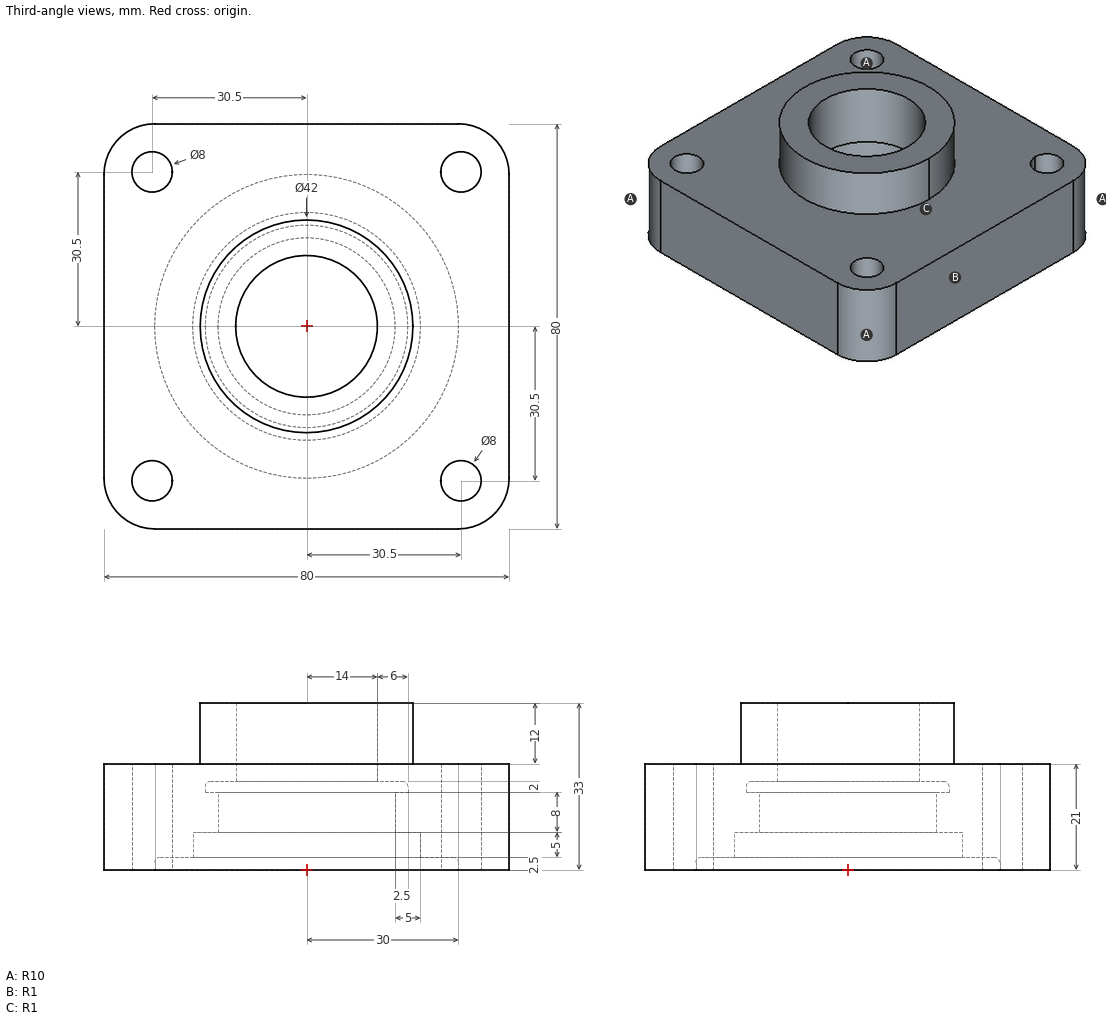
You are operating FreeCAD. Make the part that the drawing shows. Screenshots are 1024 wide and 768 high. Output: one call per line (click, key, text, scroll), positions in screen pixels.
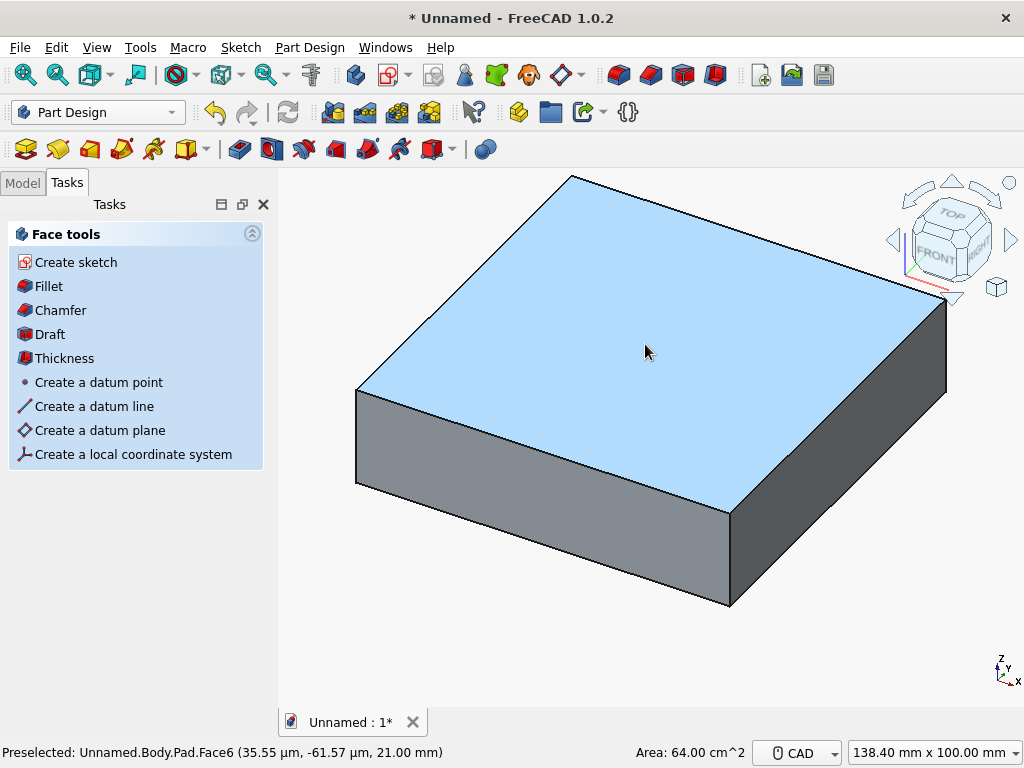
click(388, 76)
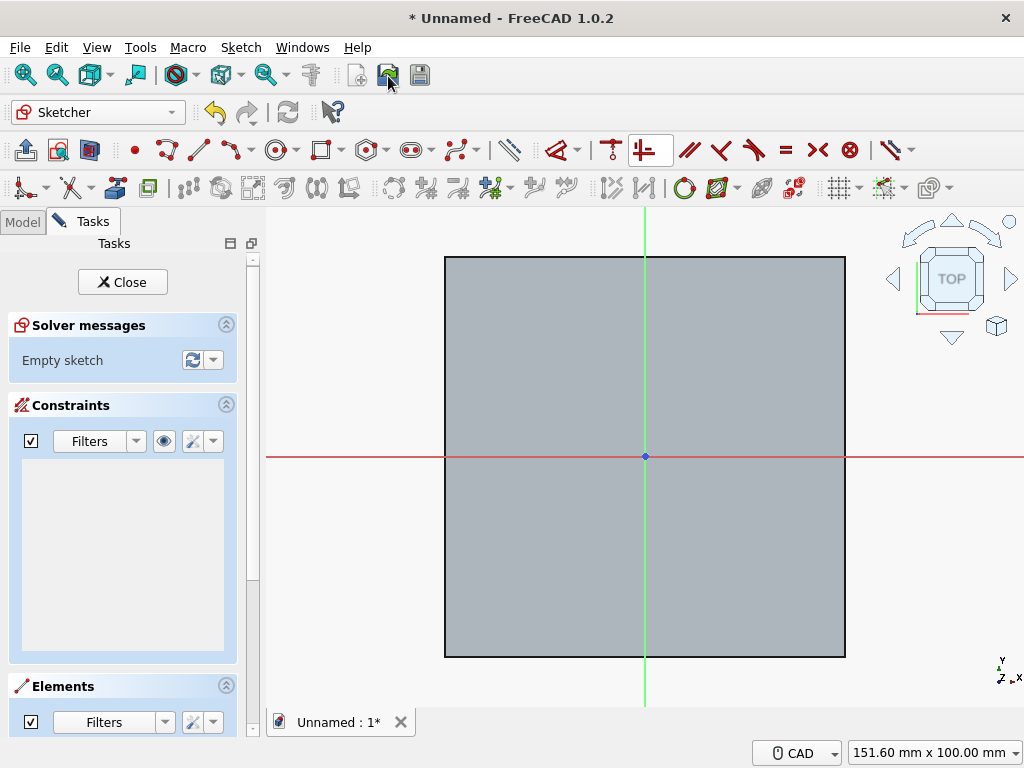
scroll(784, 457, up, 2)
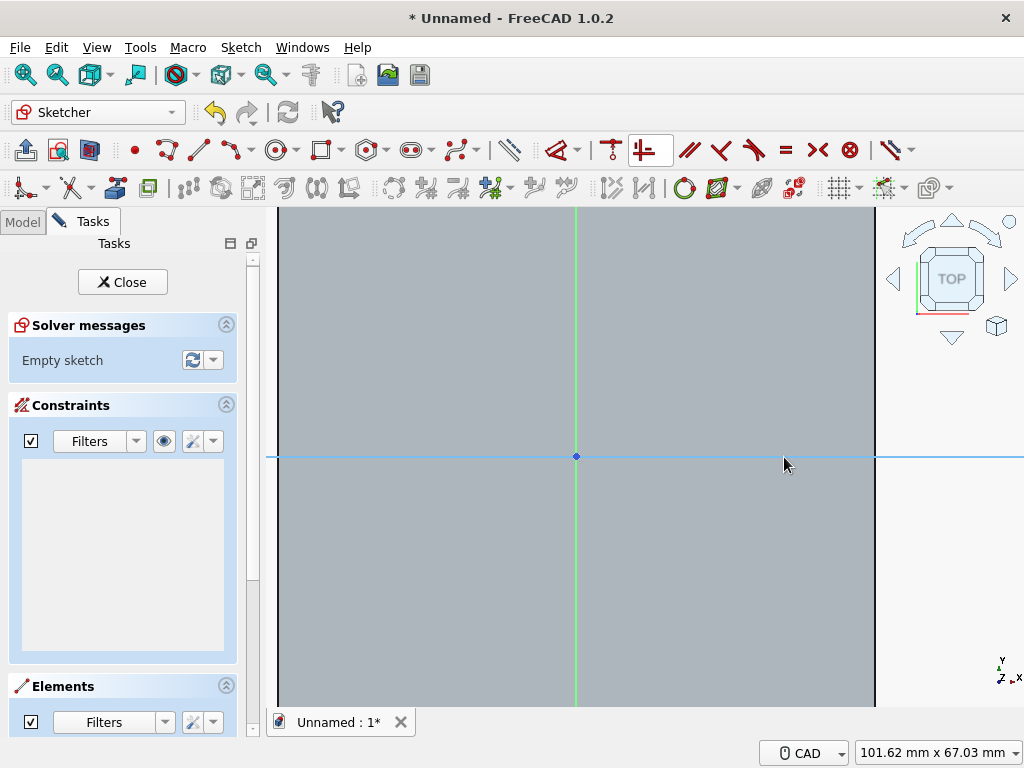
click(276, 150)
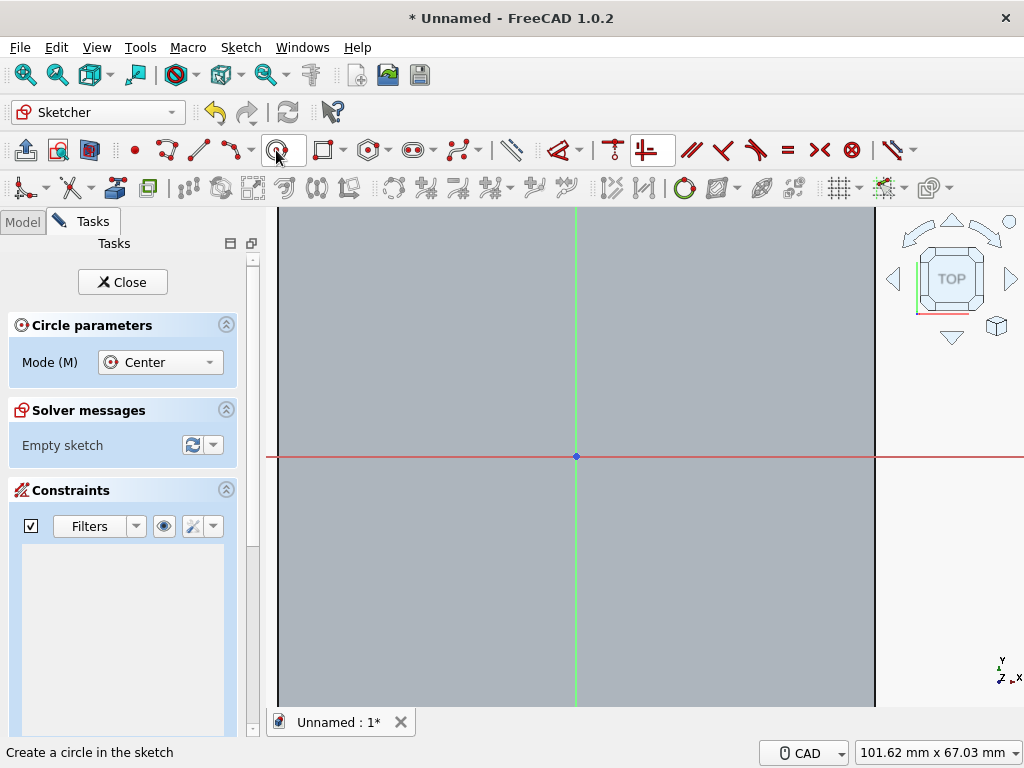
click(576, 457)
move(687, 346)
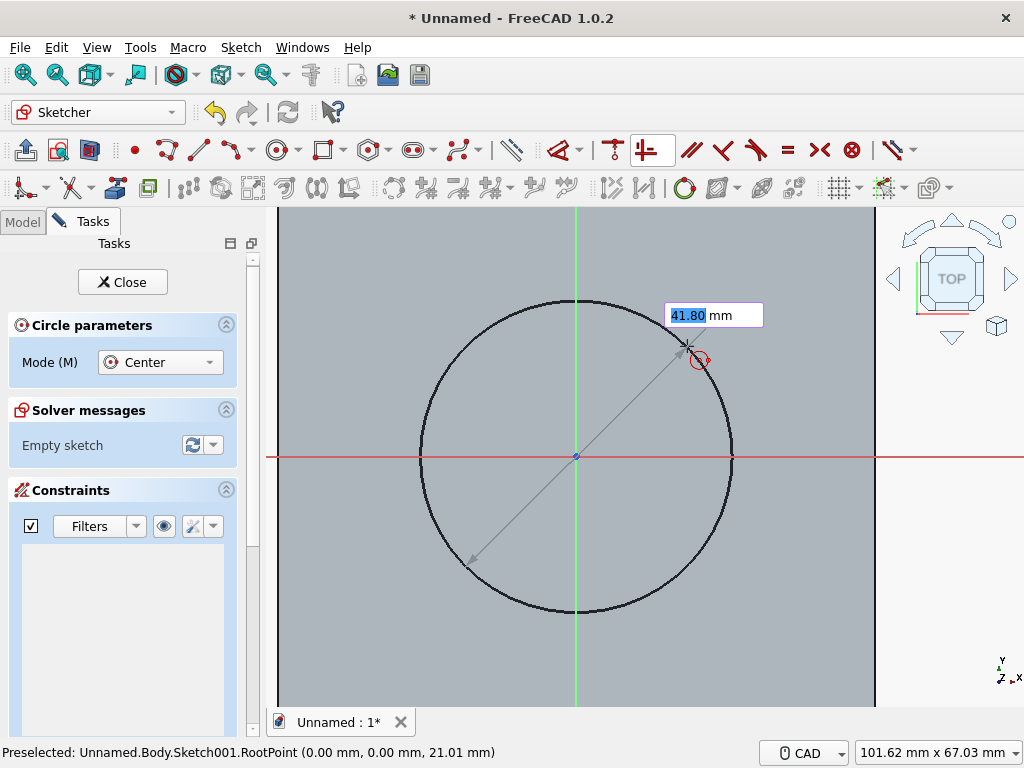
text(42)
key(Return)
key(Escape)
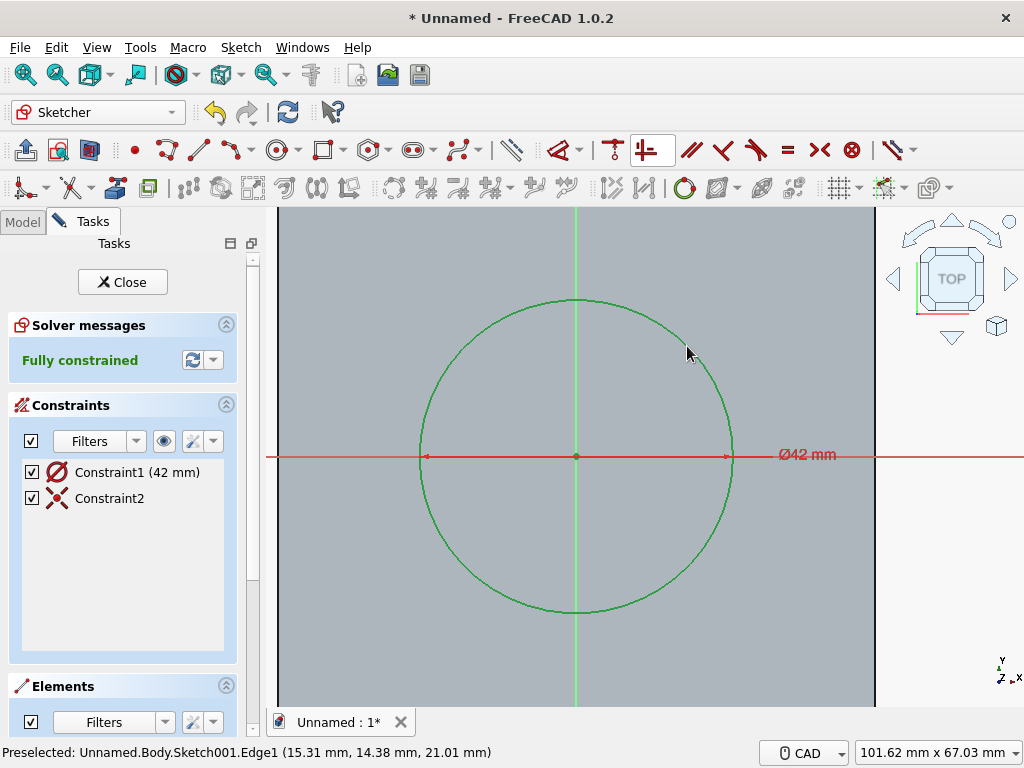
click(123, 282)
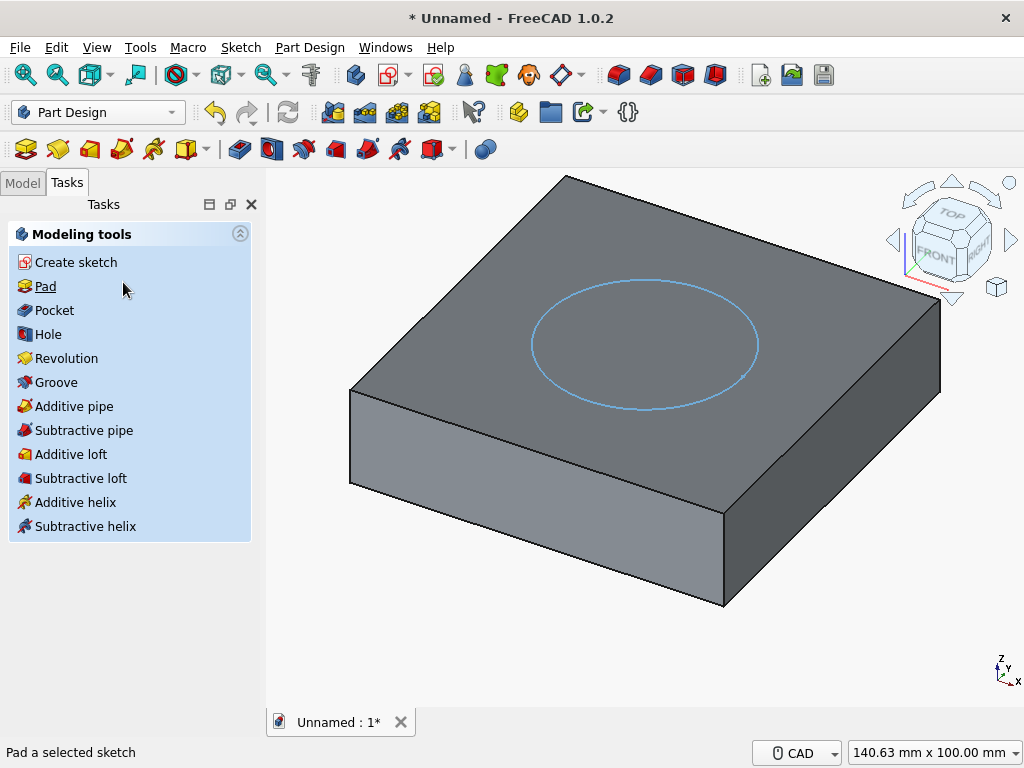
click(26, 150)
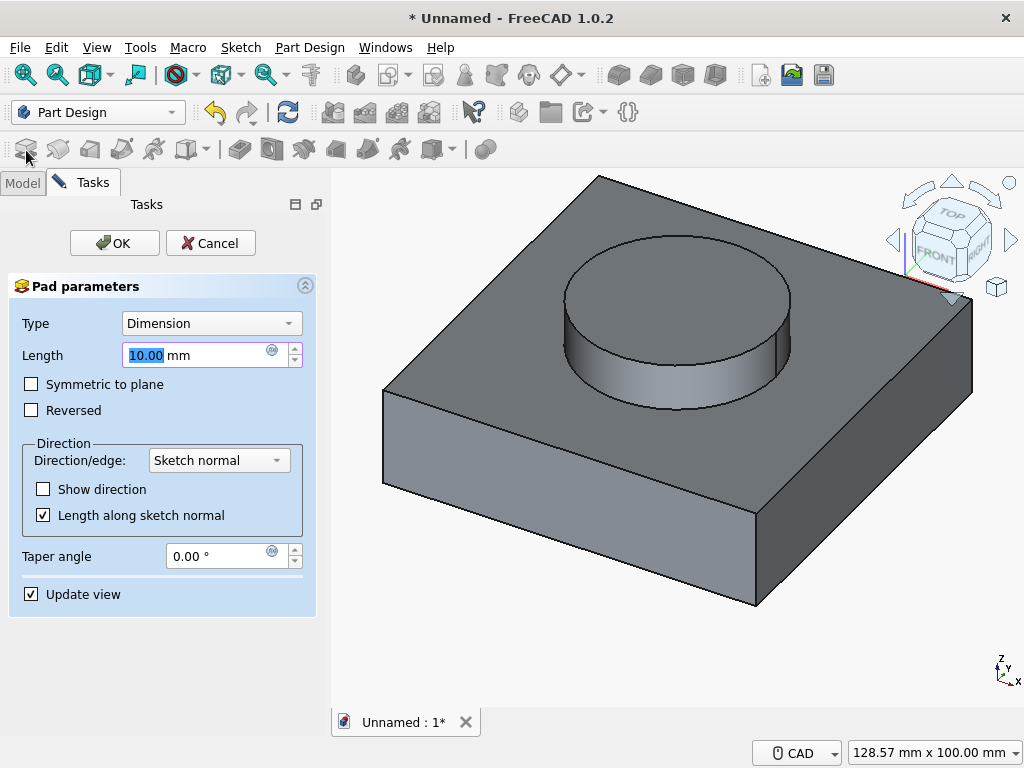
text(12)
key(Tab)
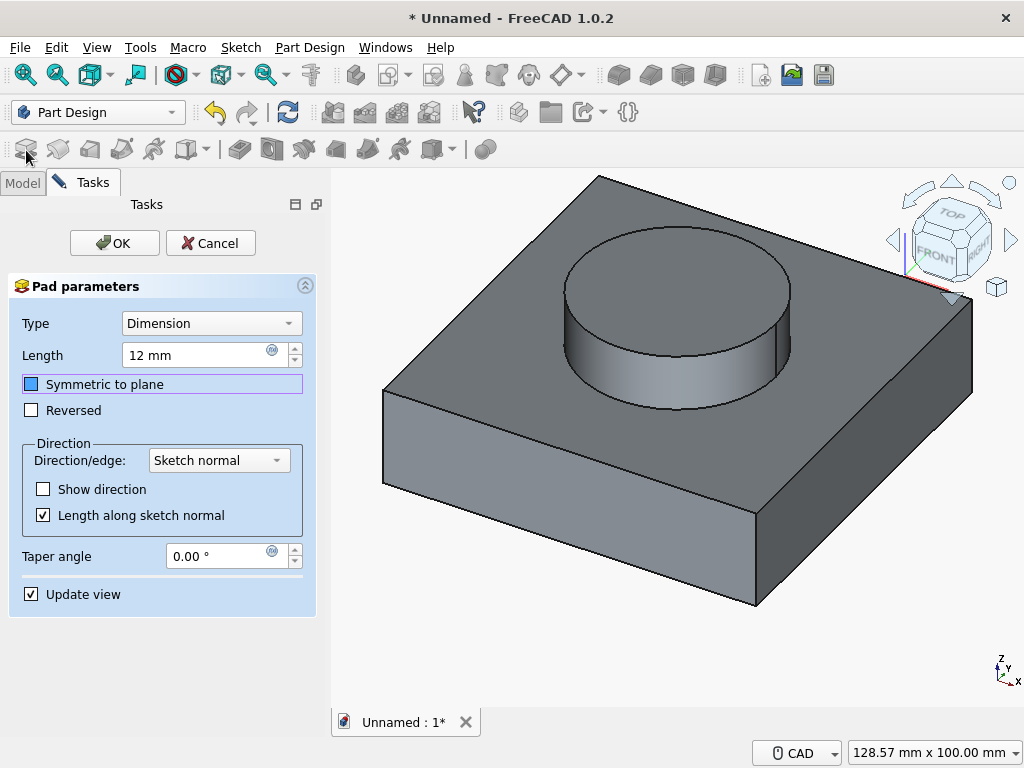
click(115, 243)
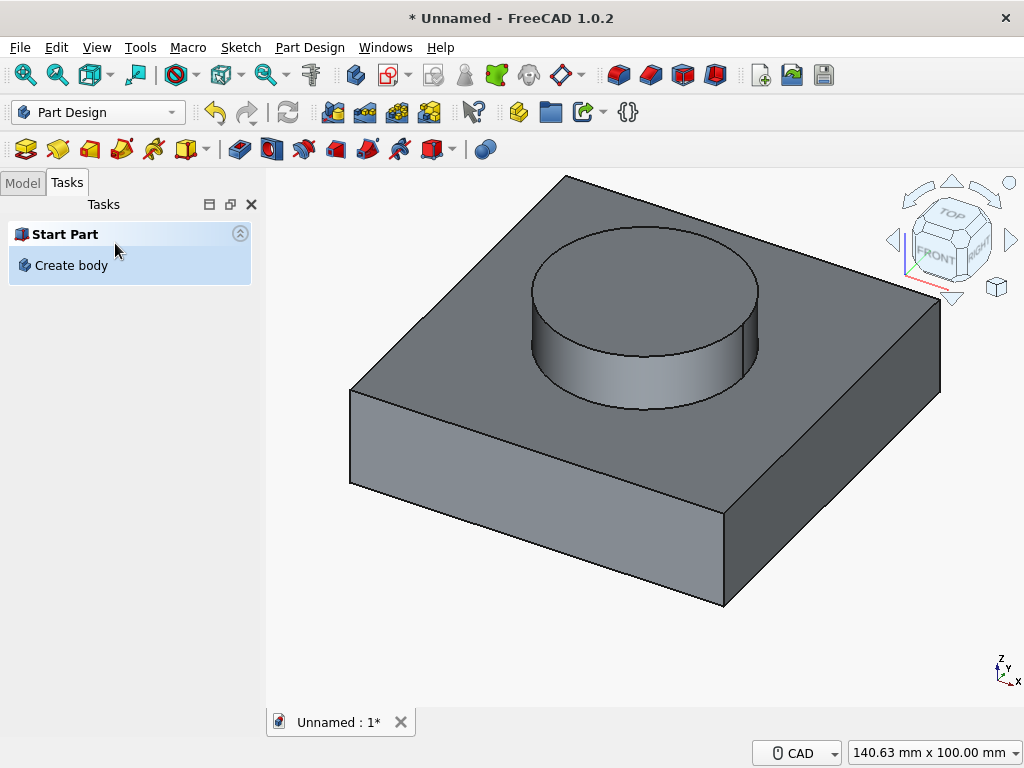
click(26, 76)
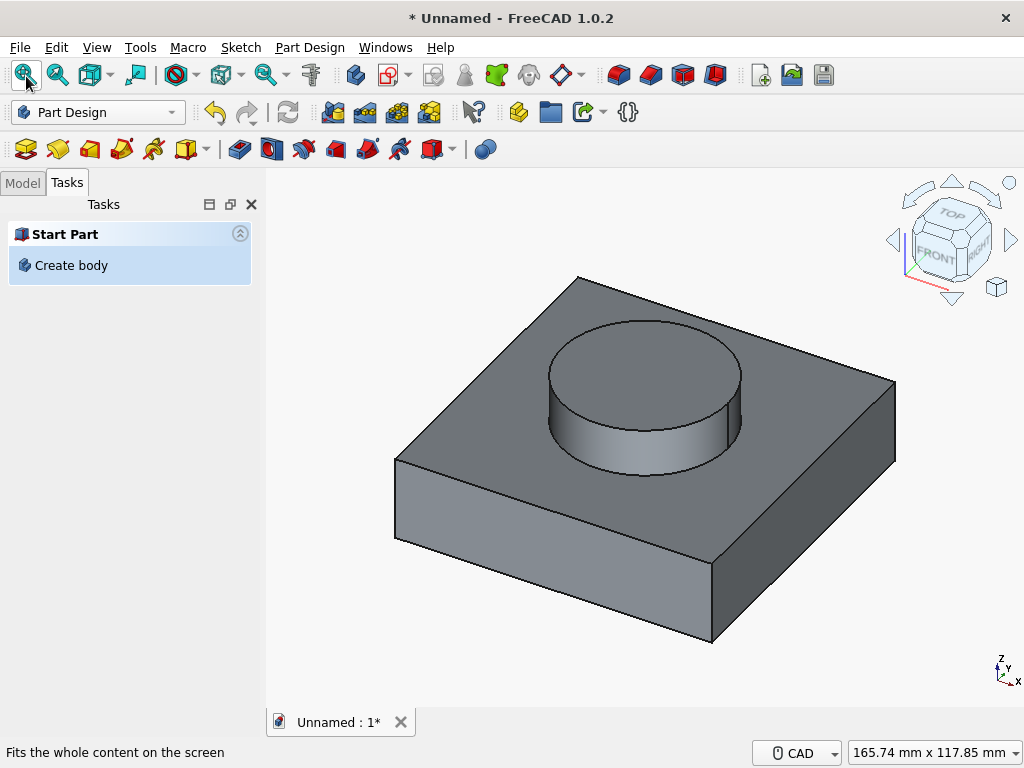
click(388, 76)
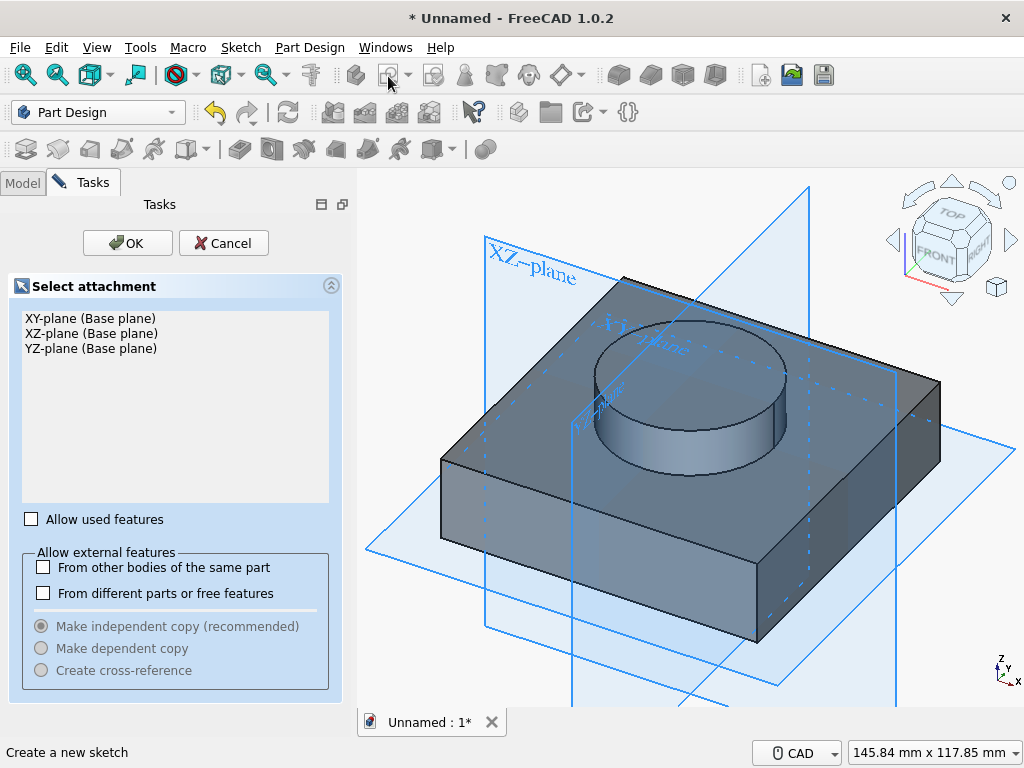
click(82, 334)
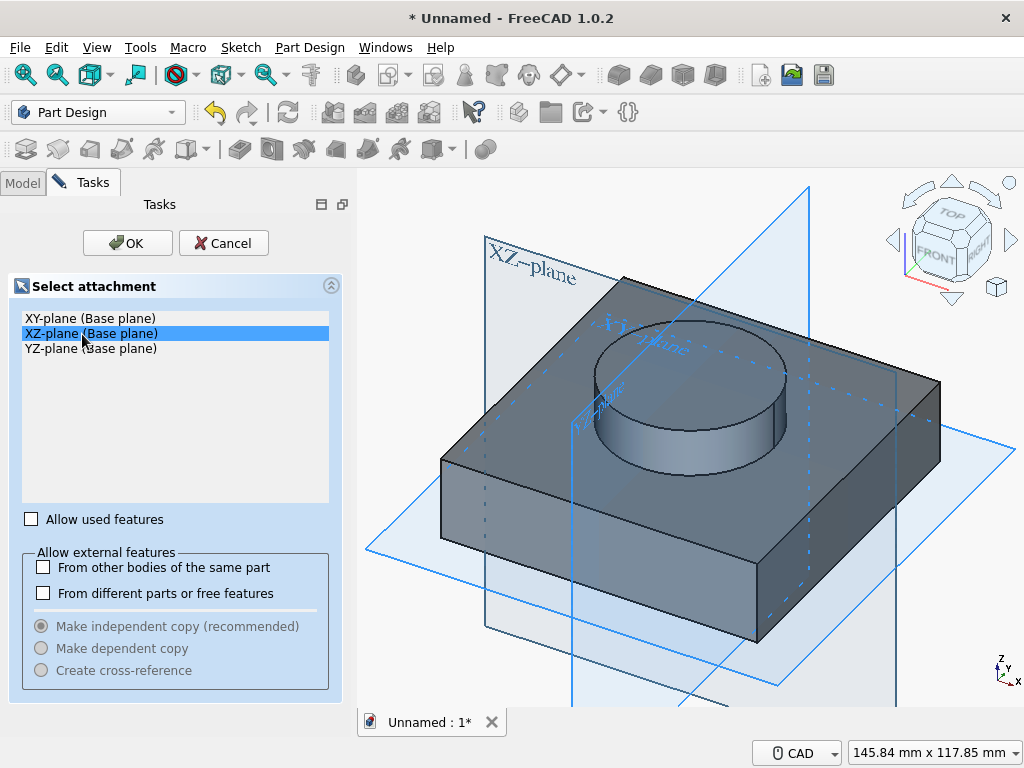
click(128, 243)